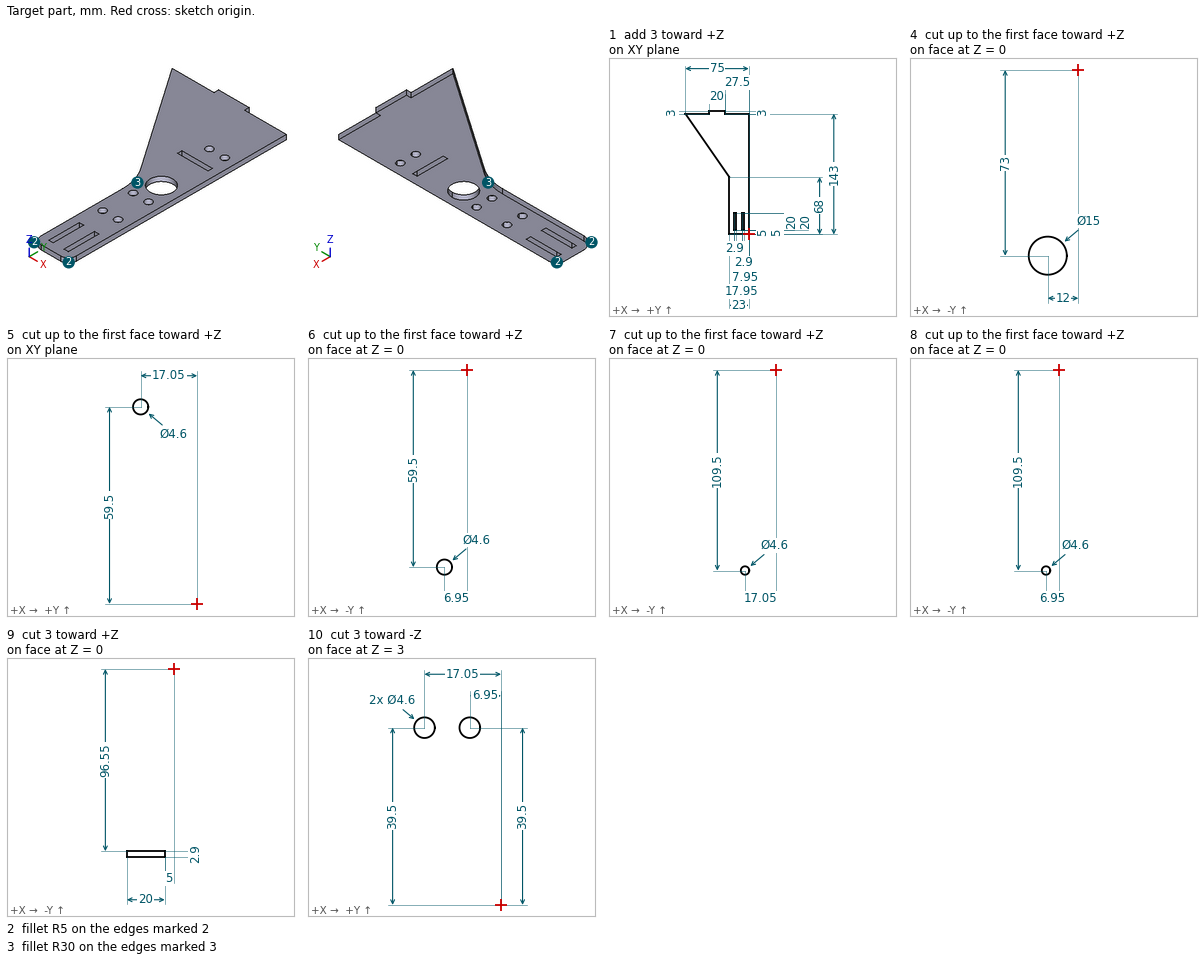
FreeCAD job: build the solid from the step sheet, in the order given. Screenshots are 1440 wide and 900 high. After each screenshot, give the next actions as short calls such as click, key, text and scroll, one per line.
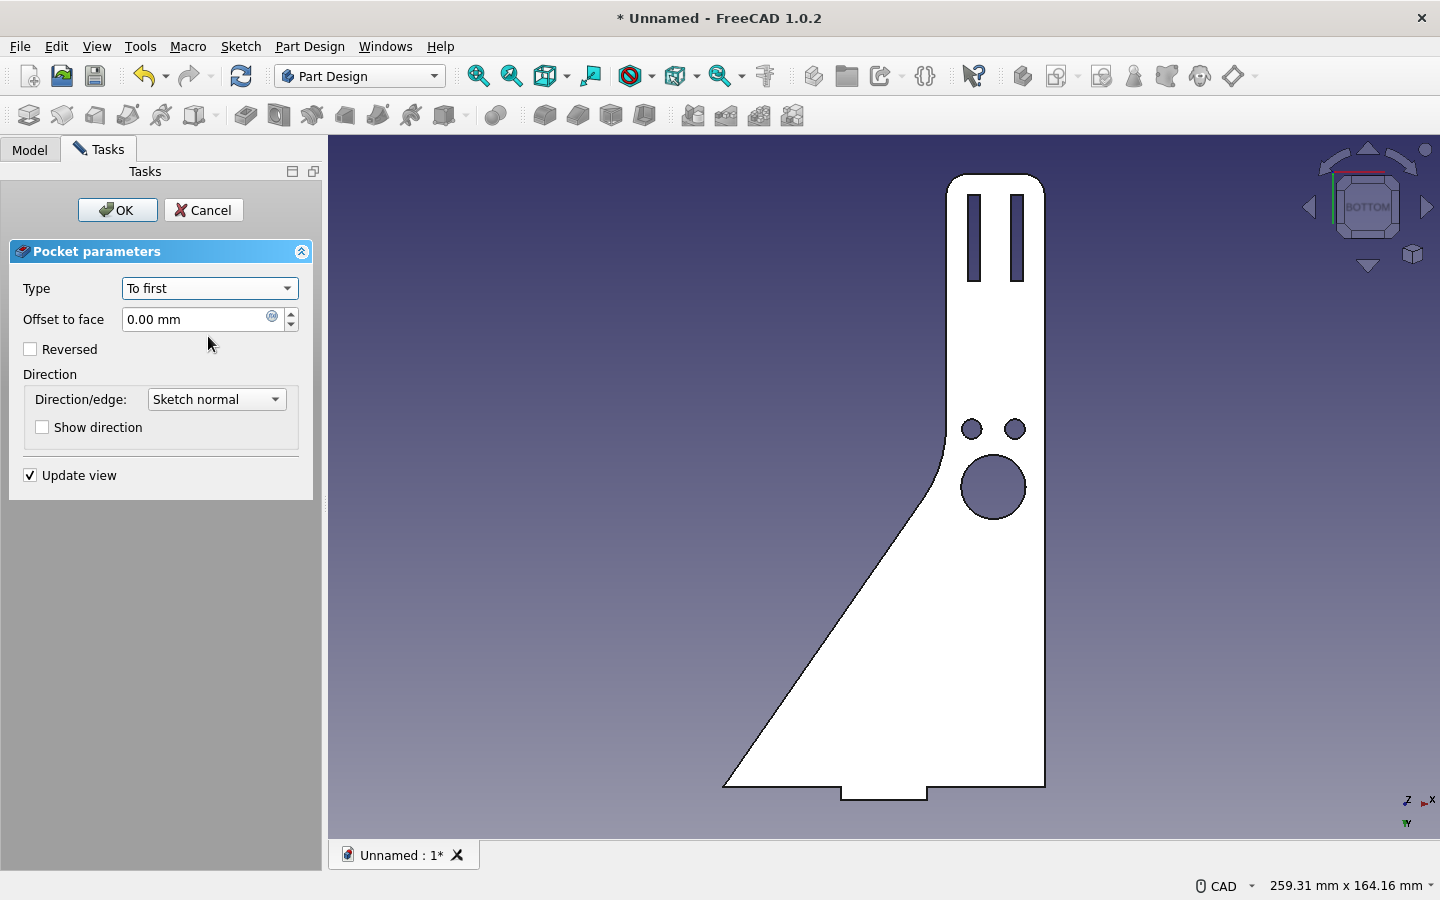
click(118, 210)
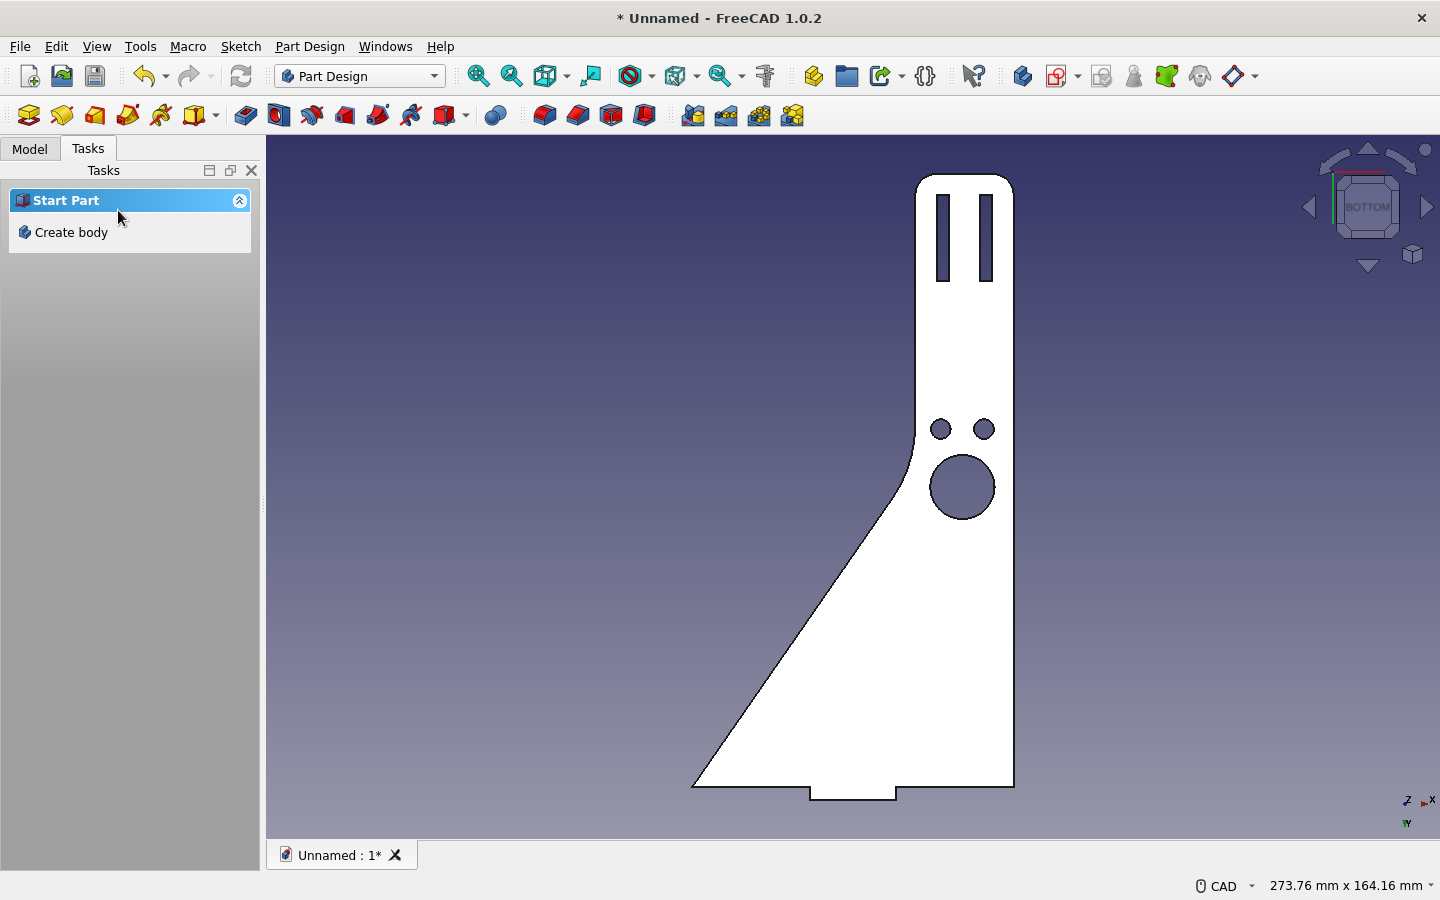
click(899, 665)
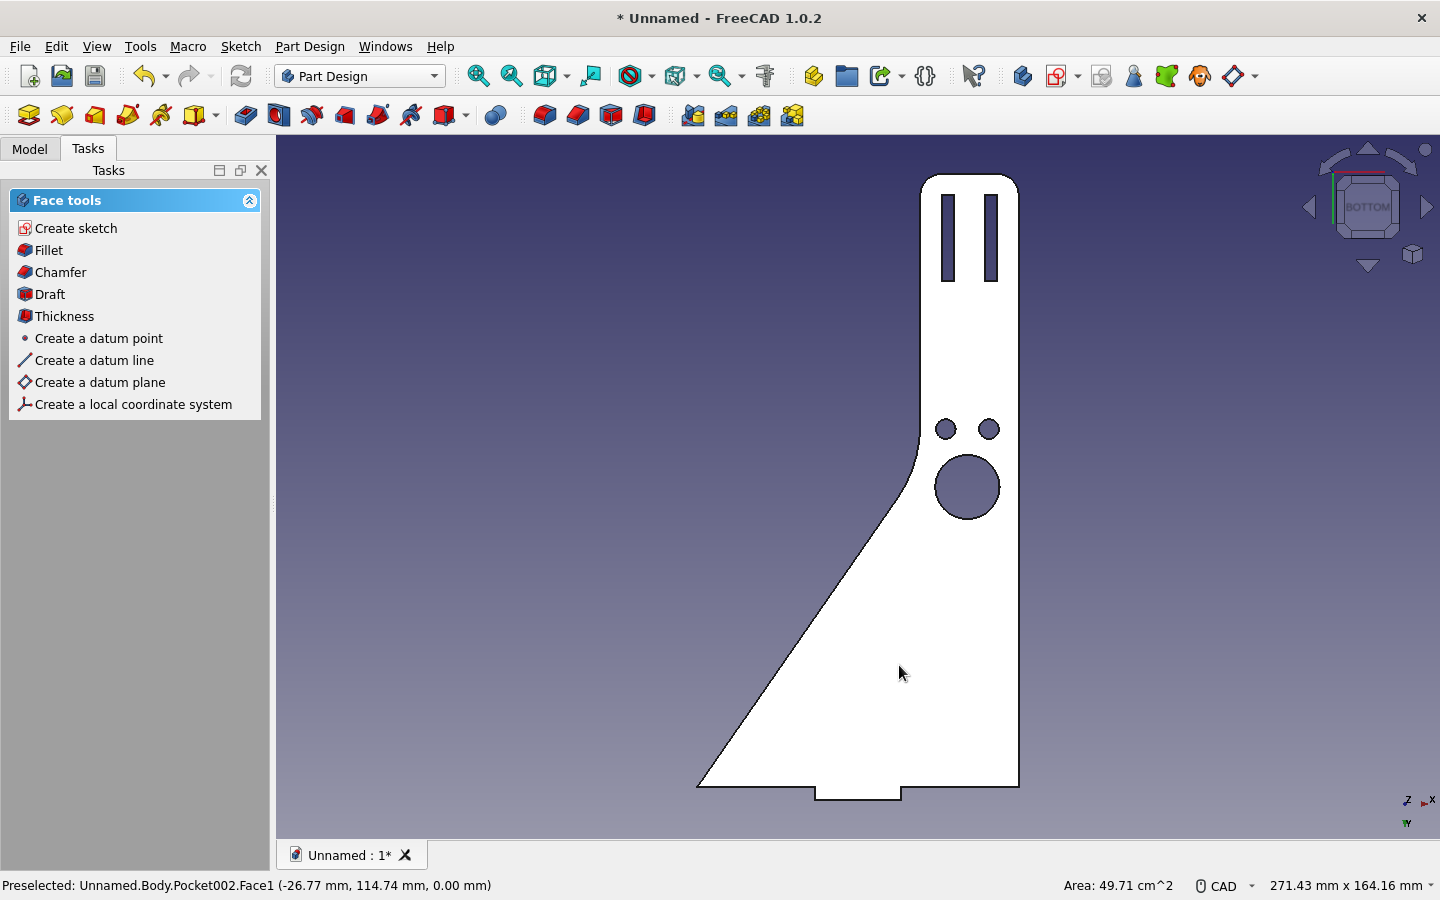
click(1056, 76)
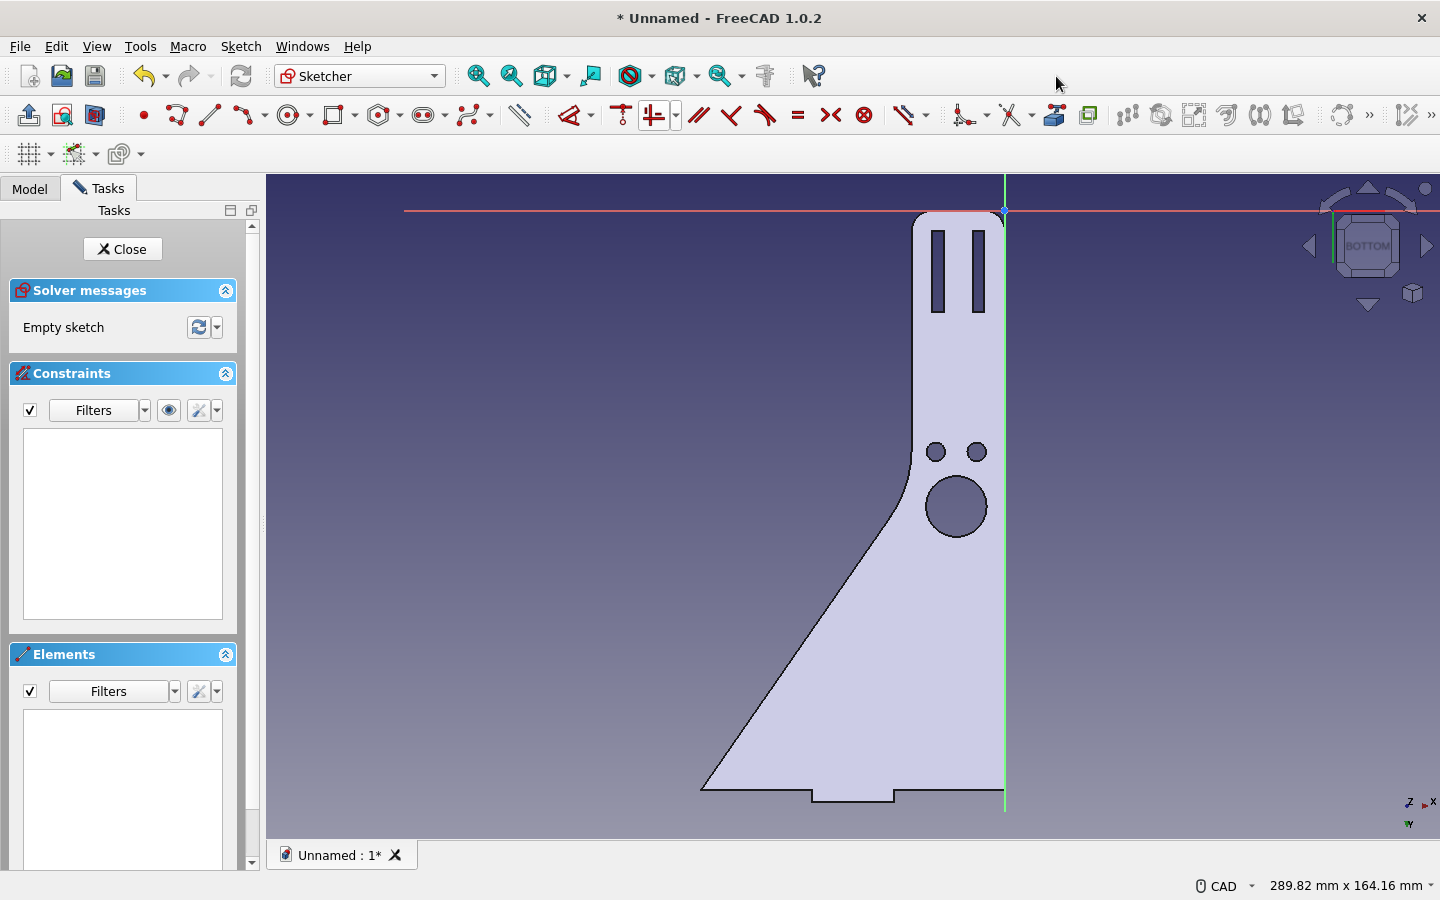
scroll(944, 662, up, 15)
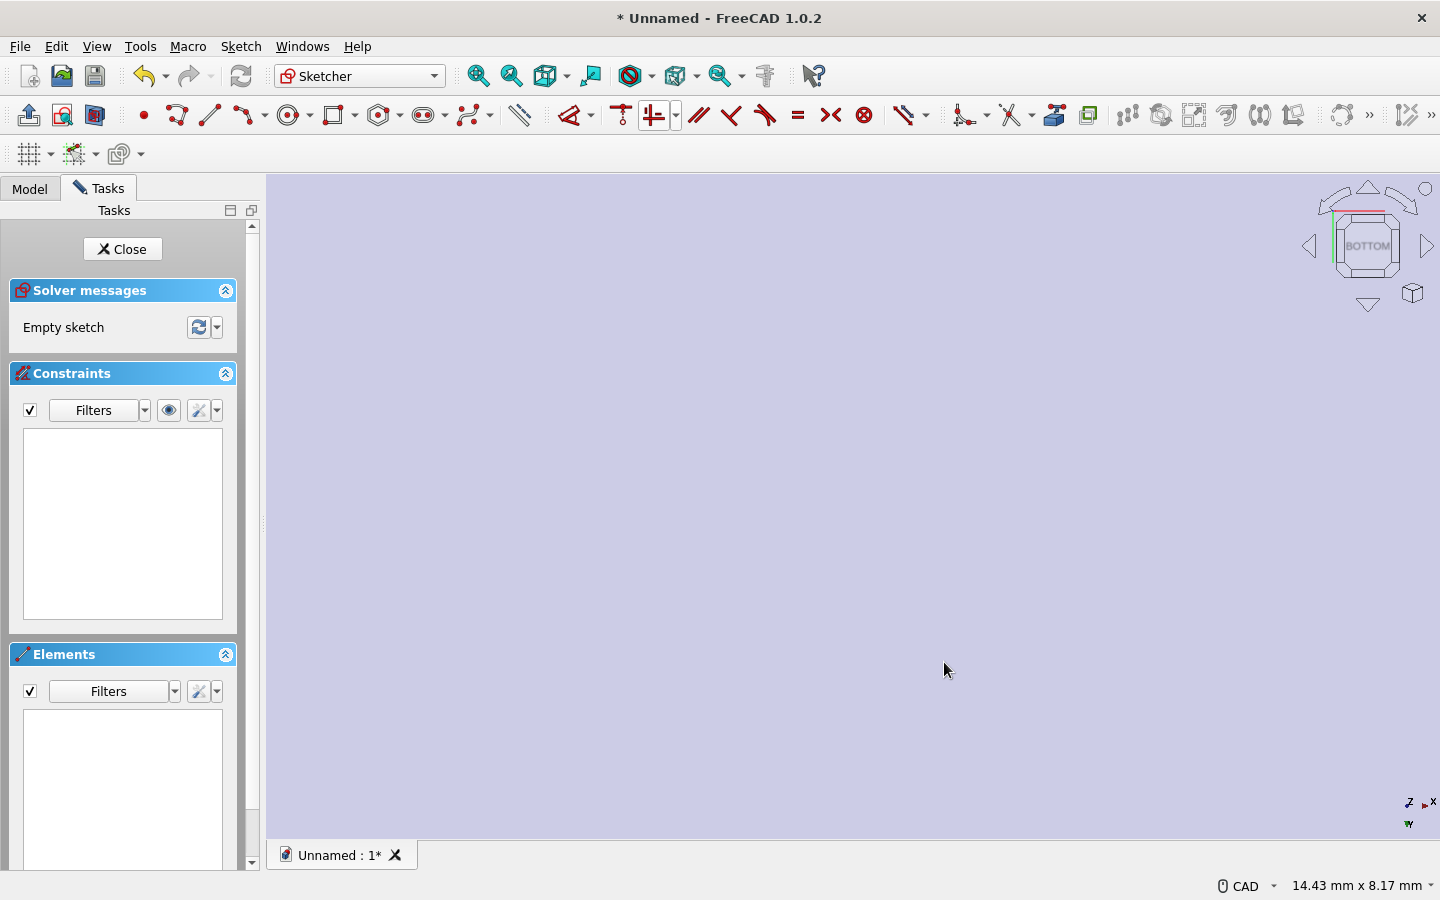
key(g)
key(c)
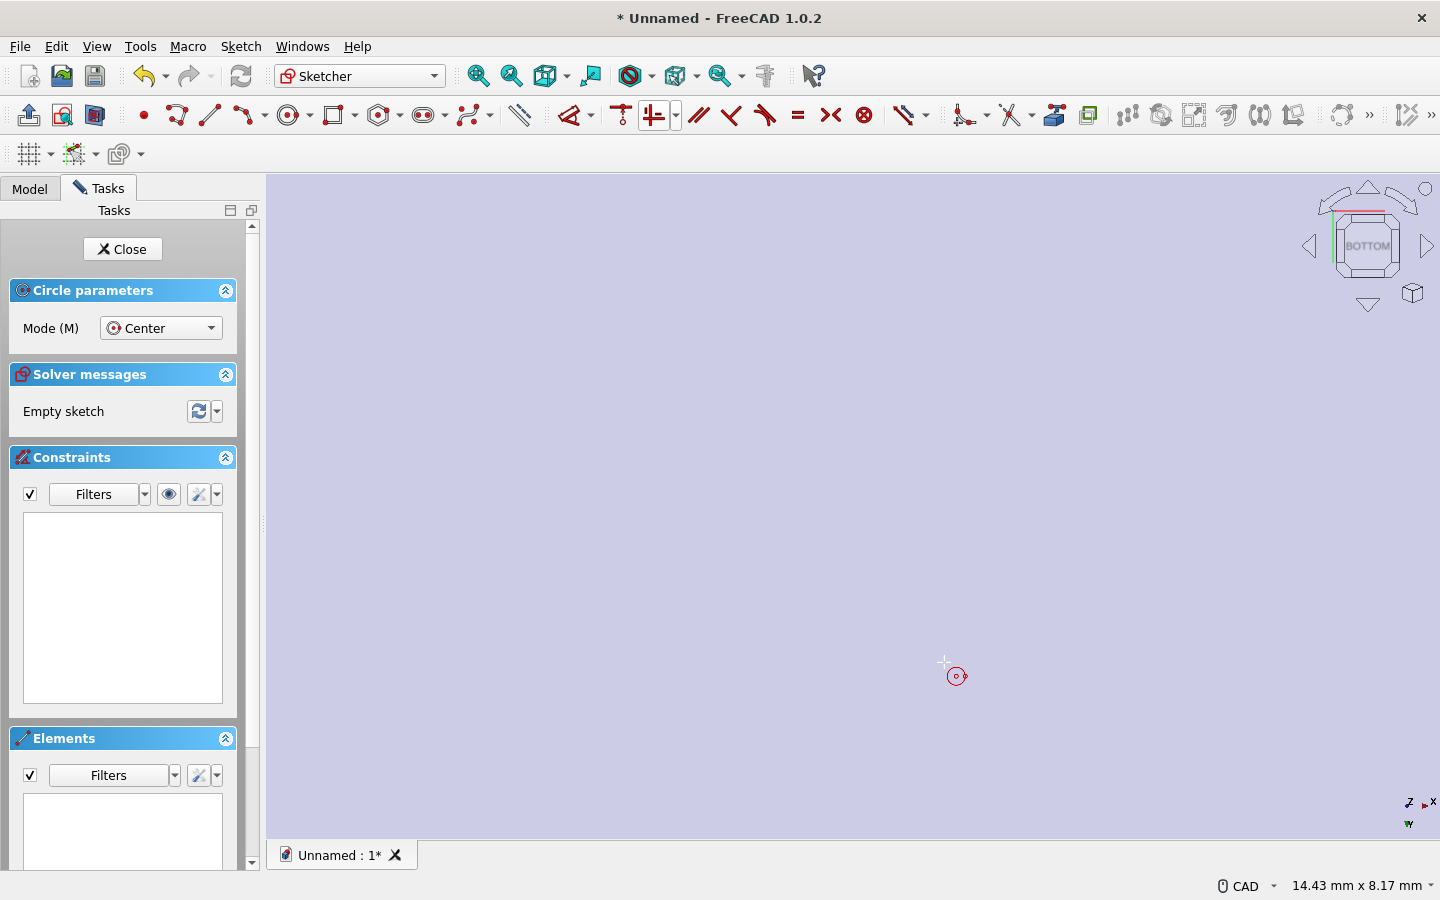
click(769, 494)
move(901, 362)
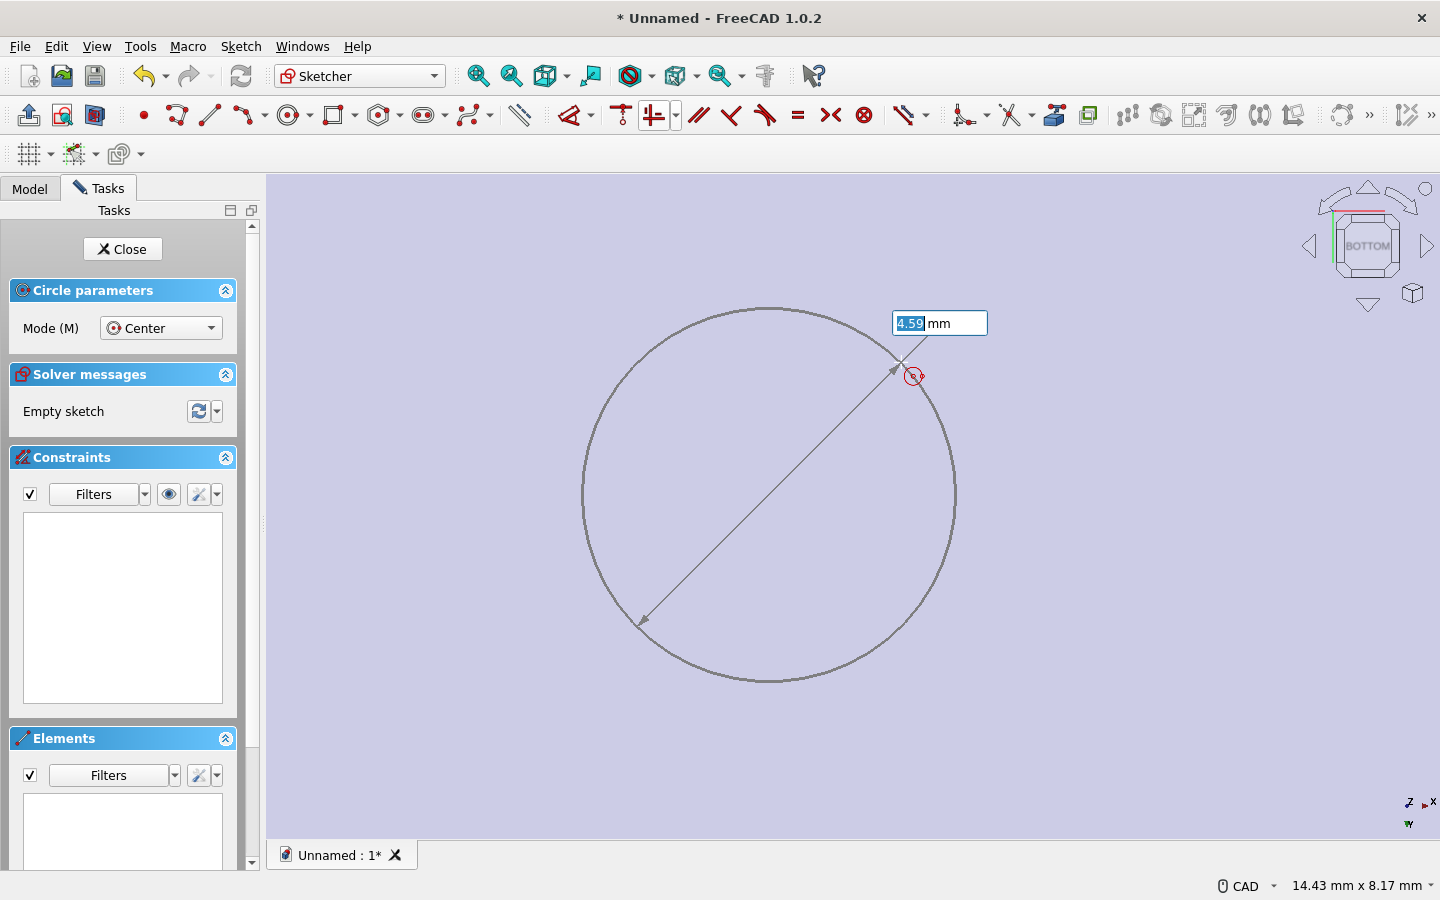
text(4.6)
key(Return)
key(Escape)